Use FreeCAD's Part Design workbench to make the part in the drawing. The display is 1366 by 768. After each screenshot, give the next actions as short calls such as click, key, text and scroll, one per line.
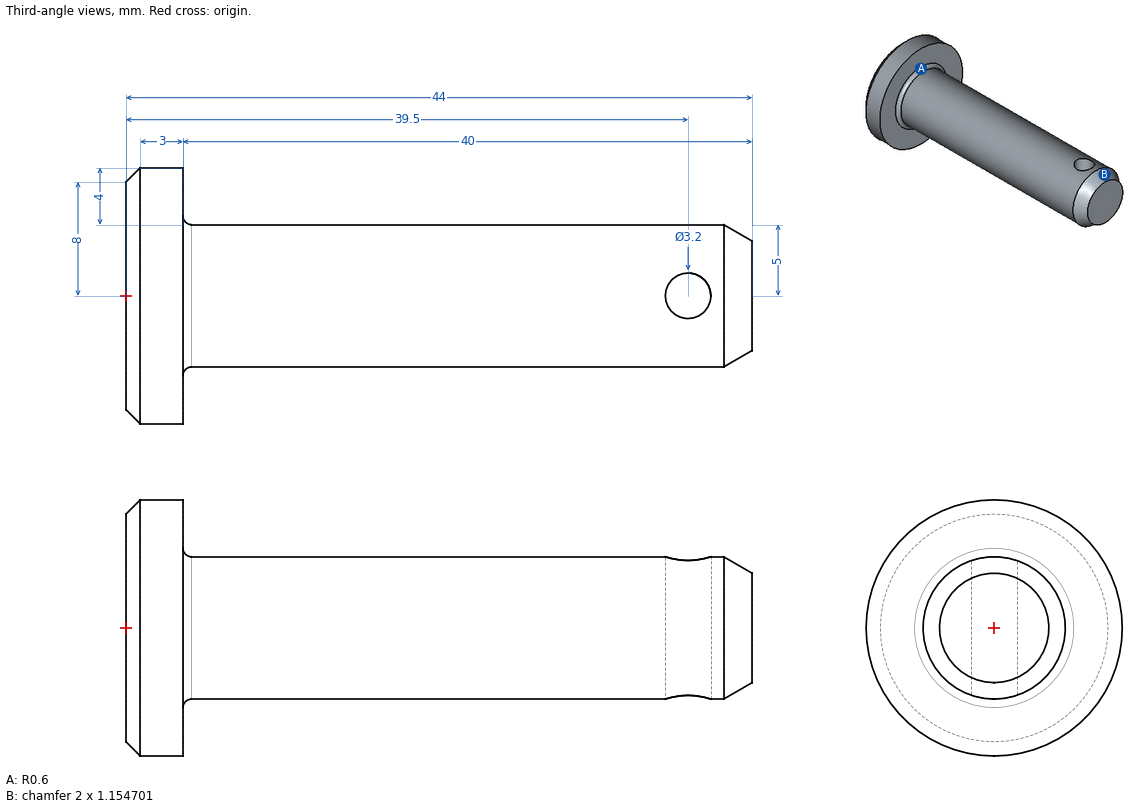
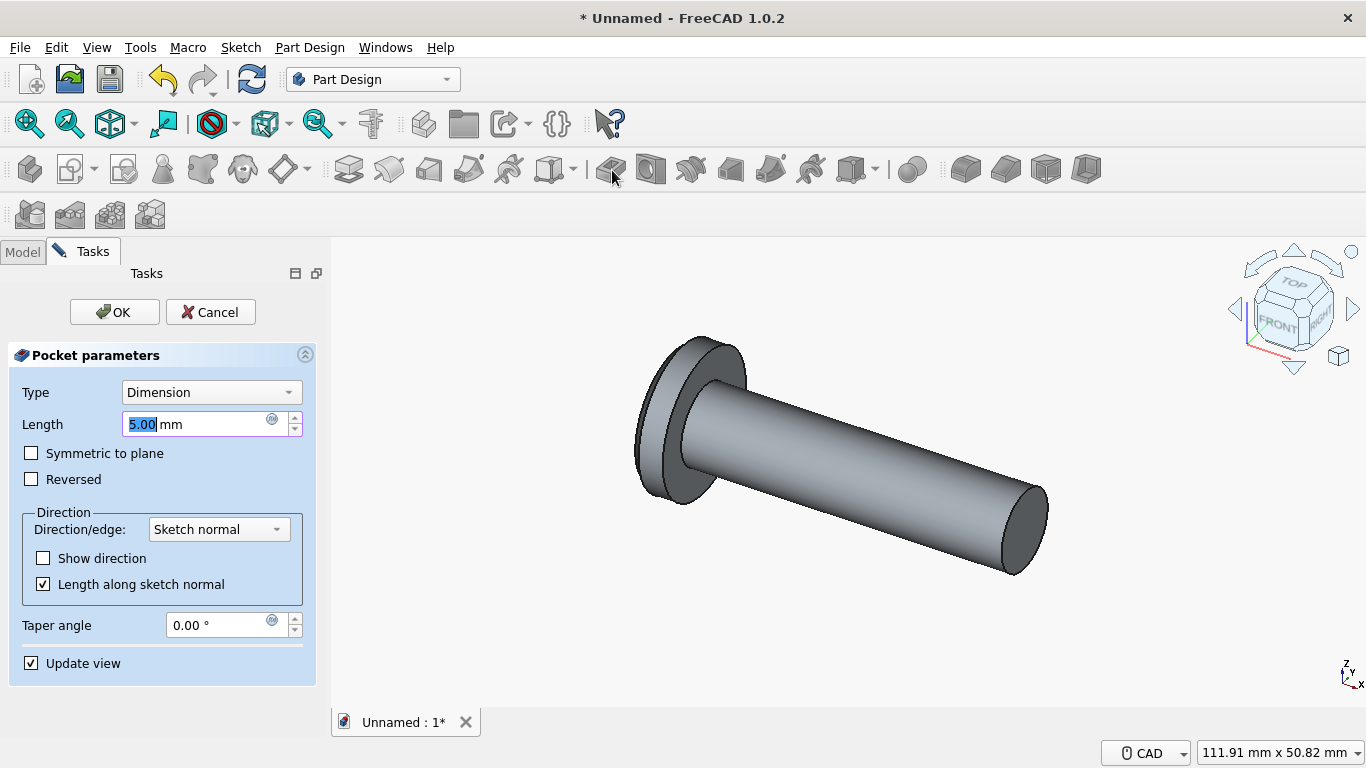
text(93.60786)
key(Tab)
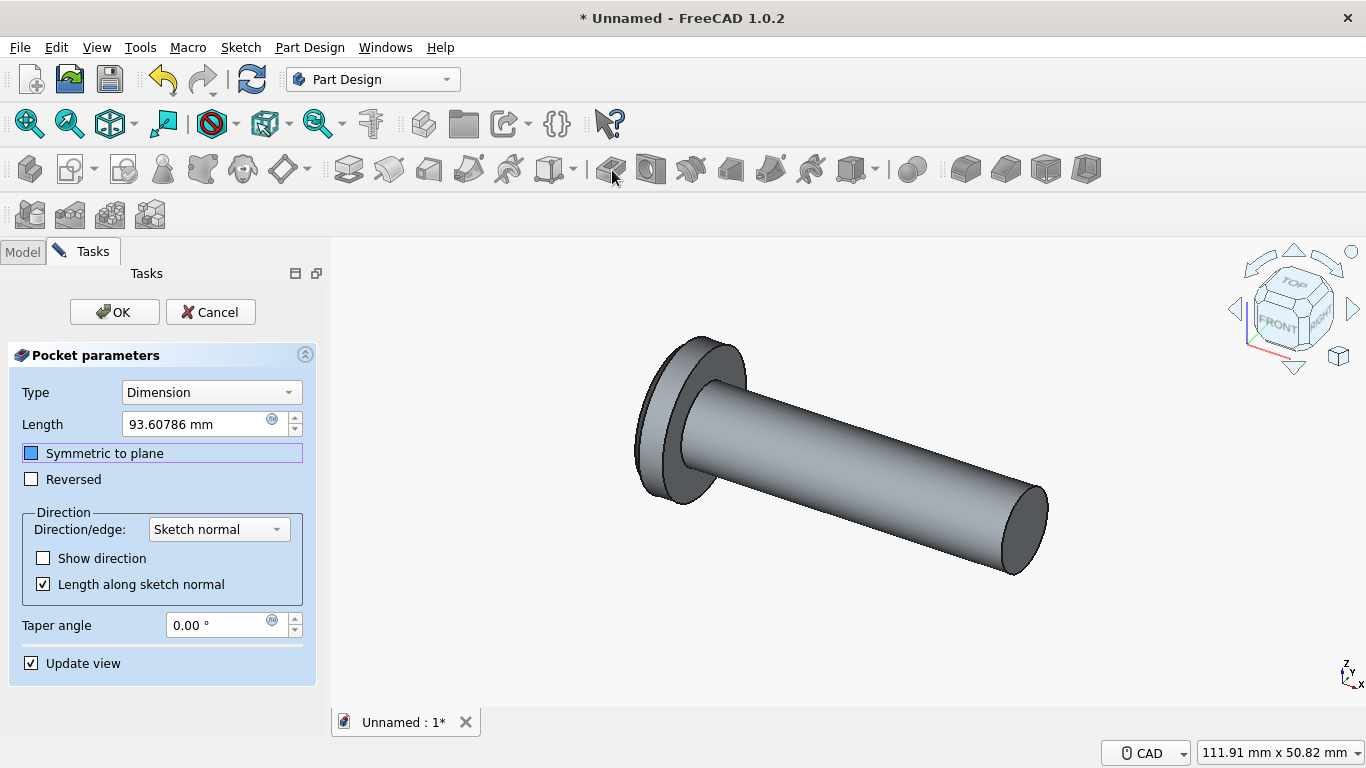
click(30, 453)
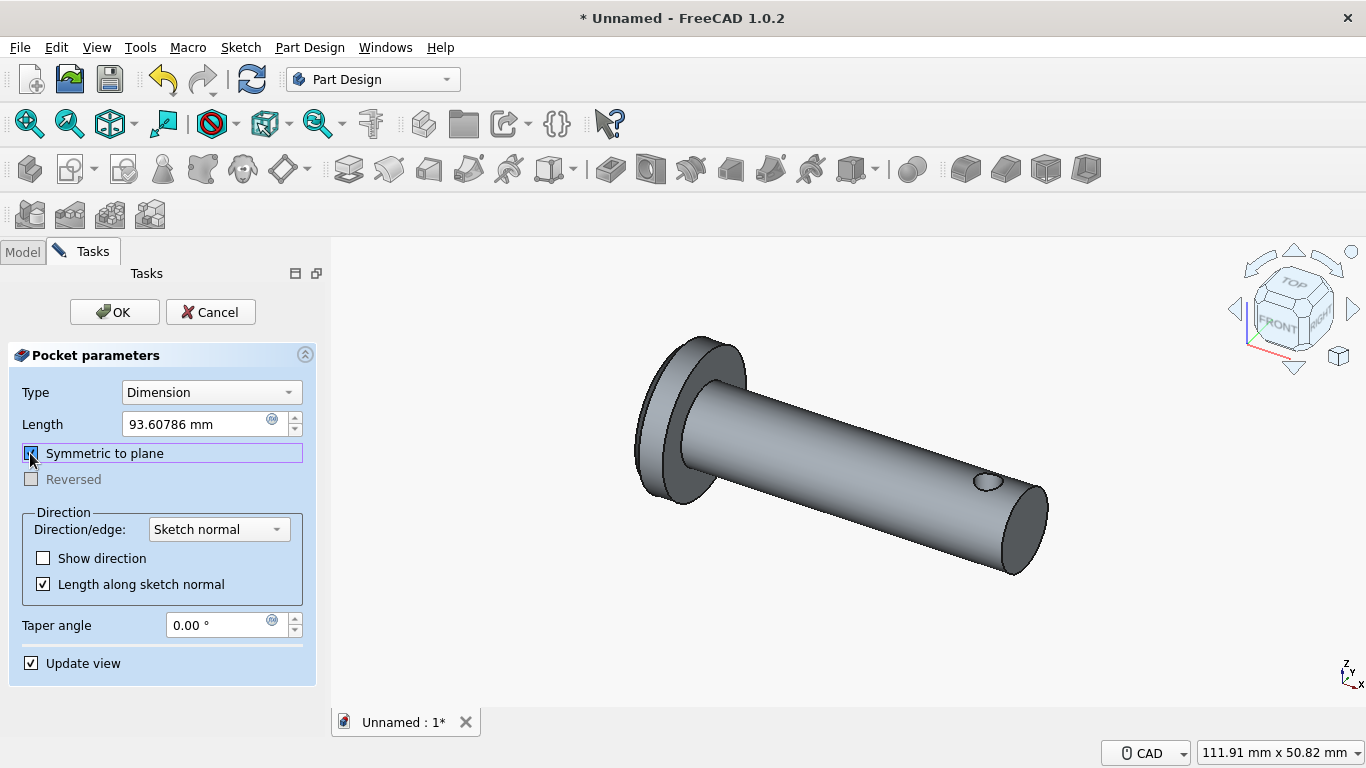
click(115, 312)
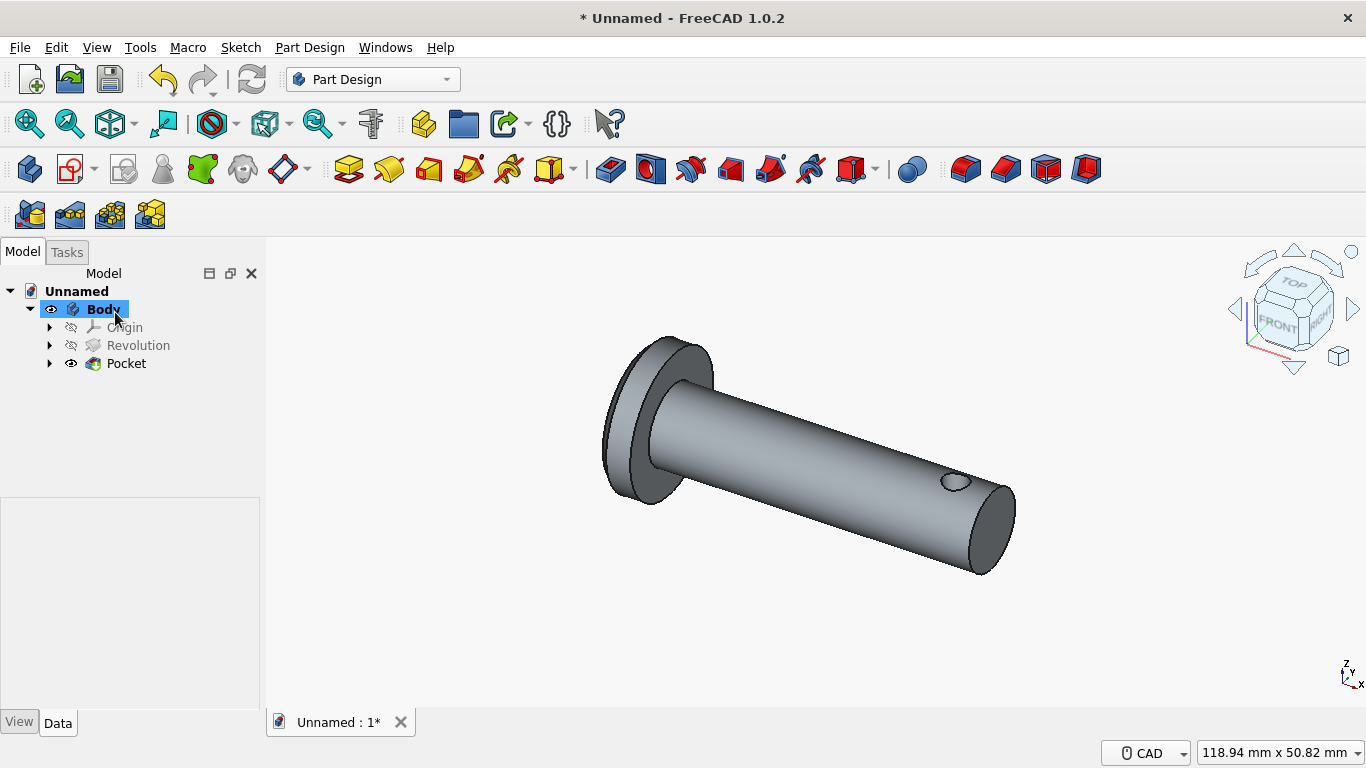
key(0)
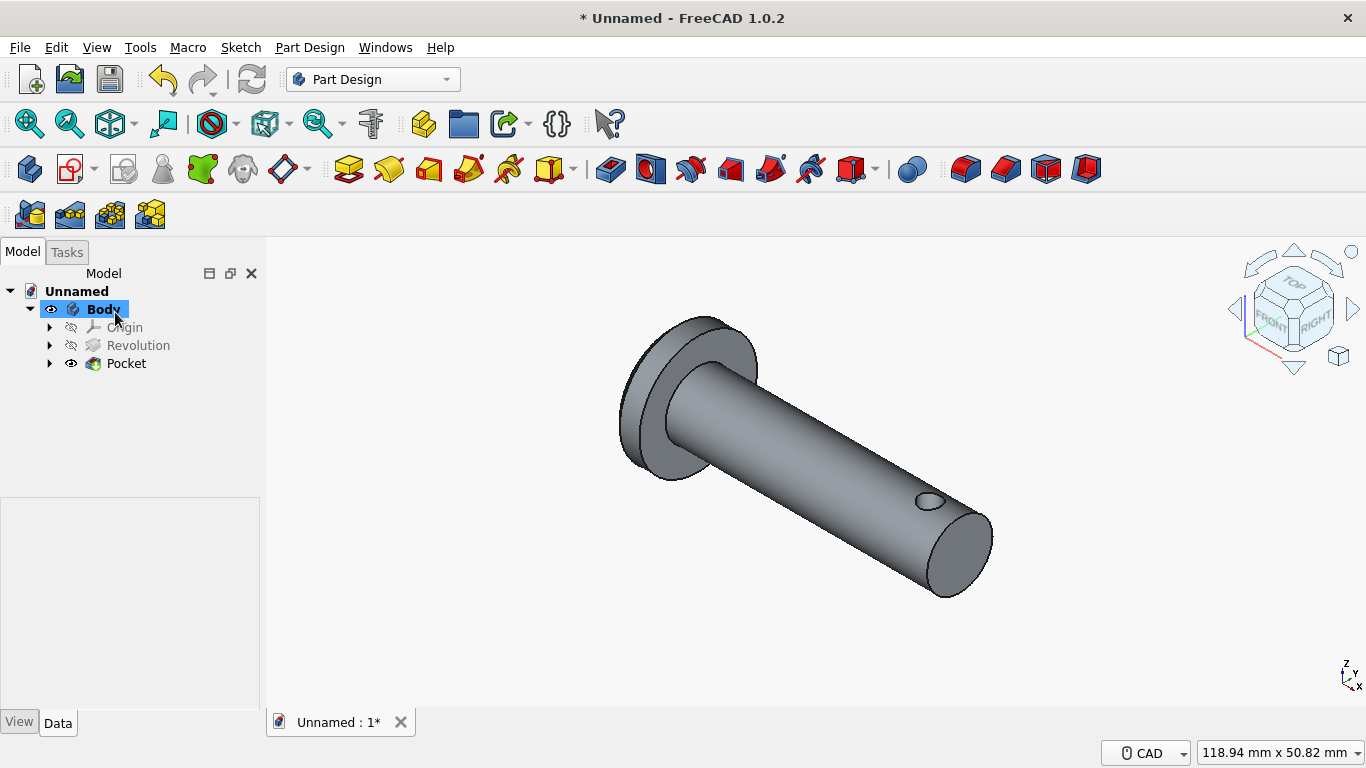
key(2)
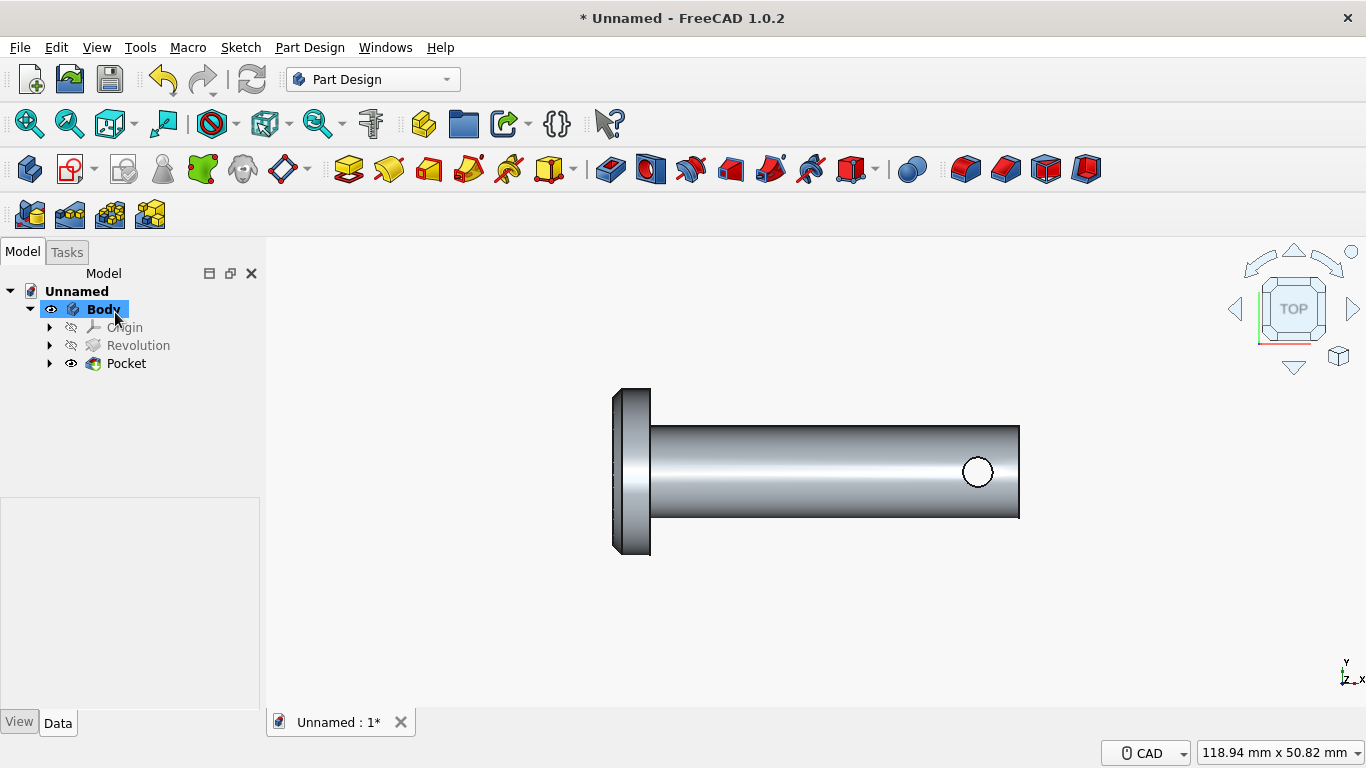
click(30, 124)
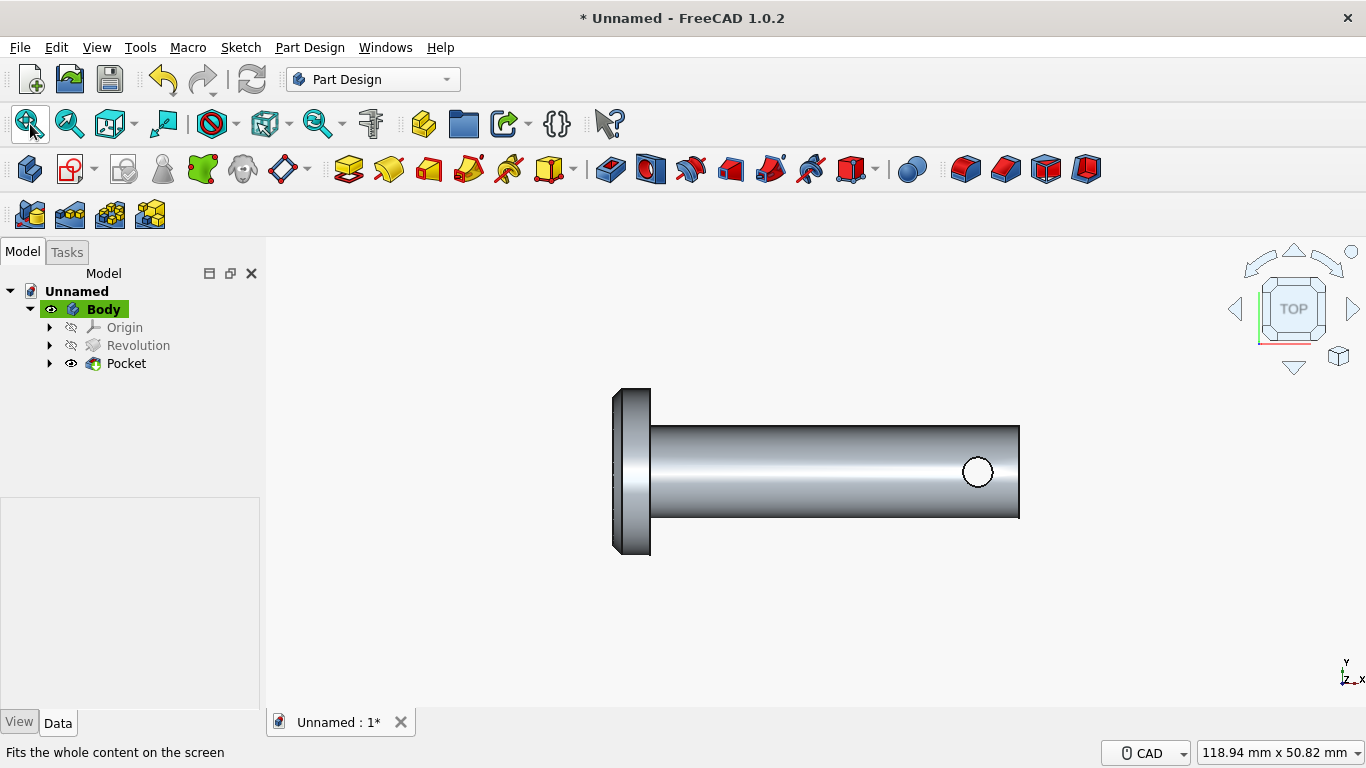
key(1)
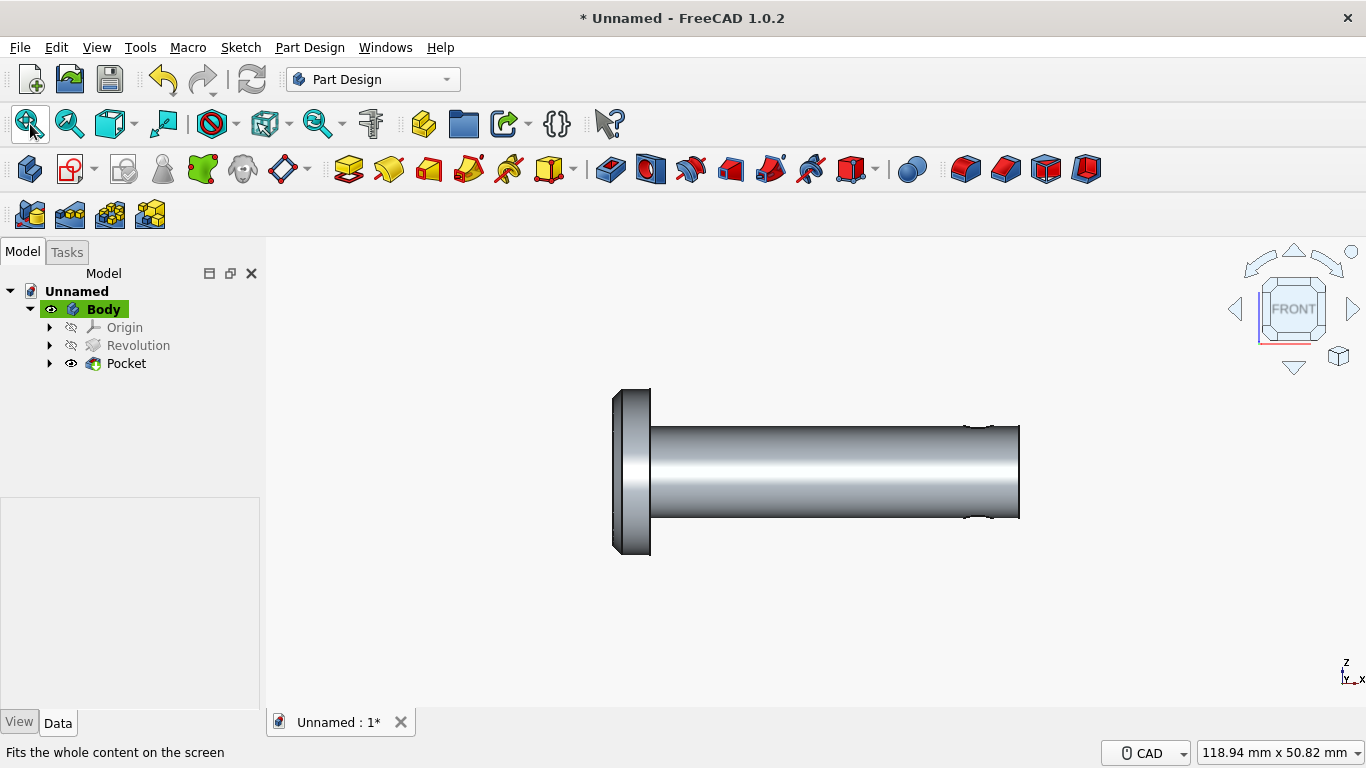
click(30, 124)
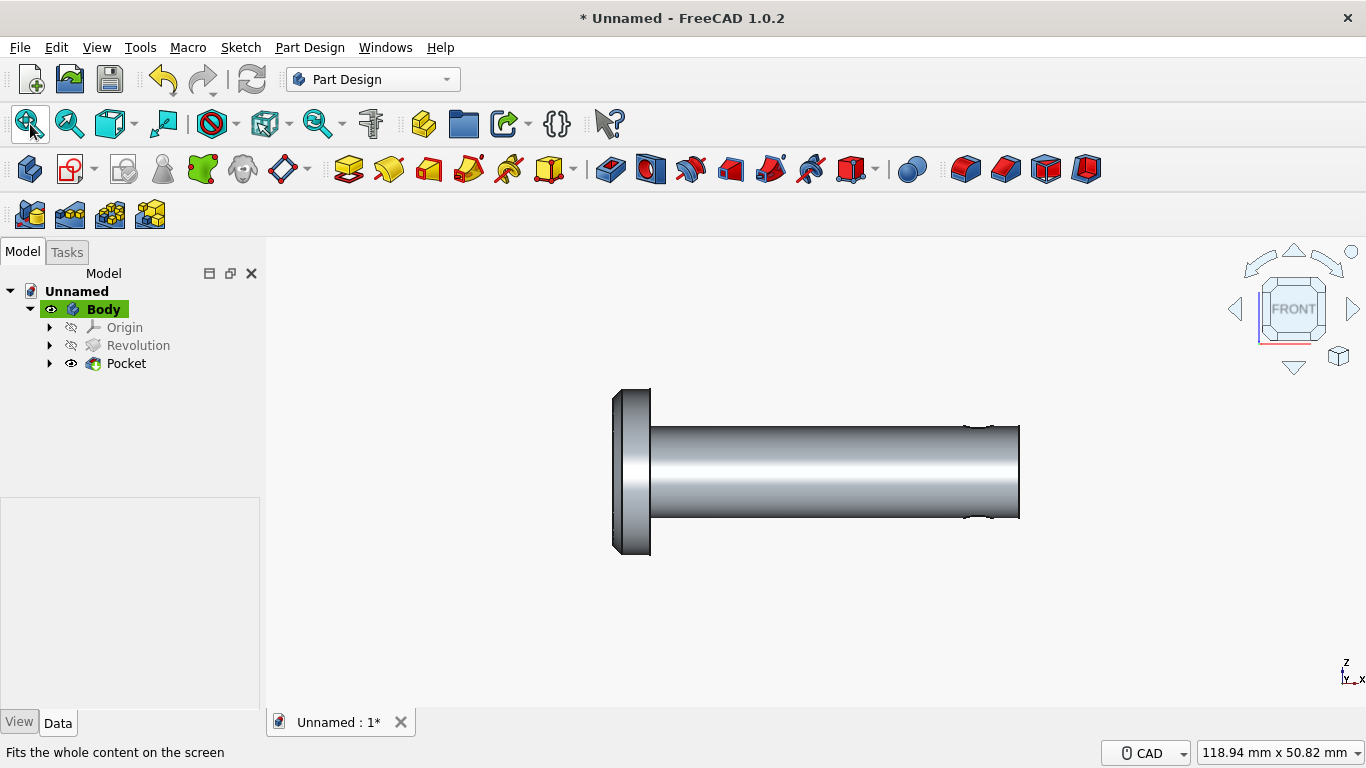
key(3)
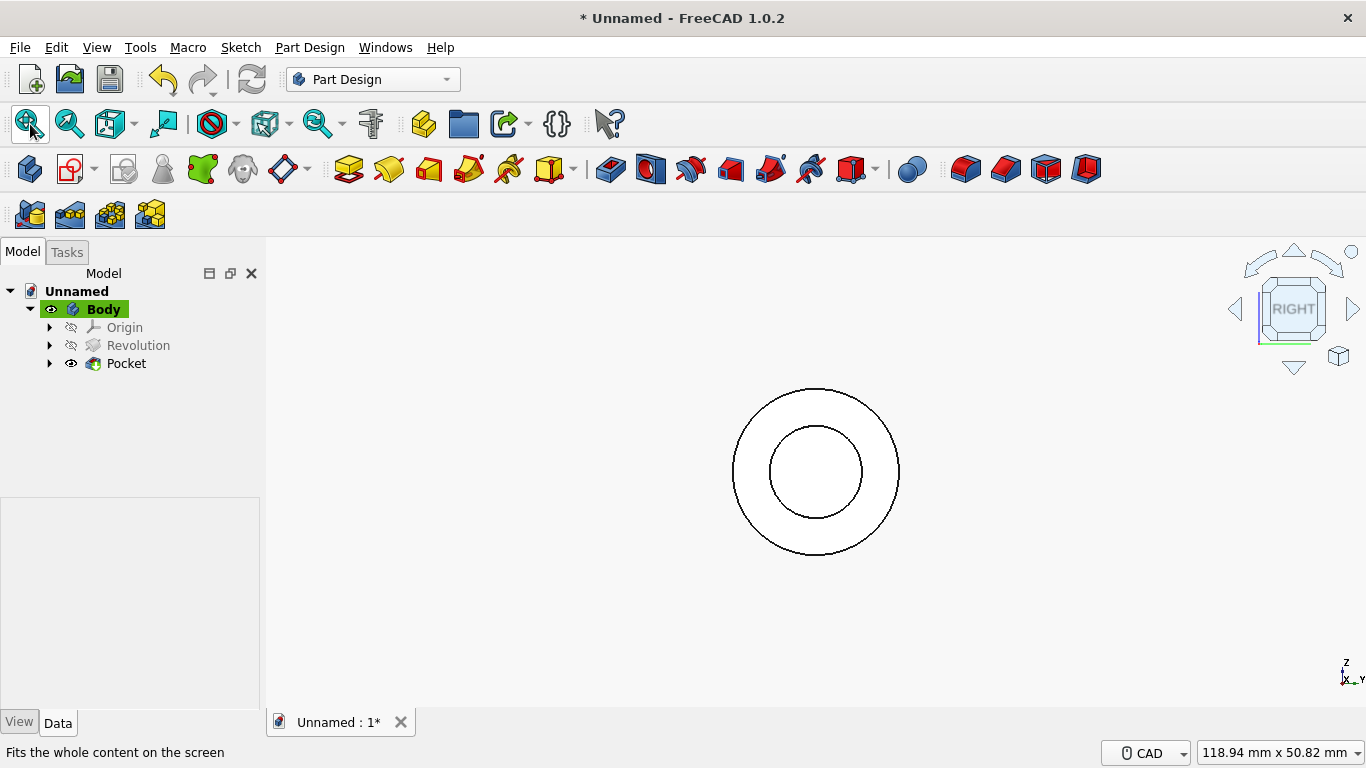
click(30, 124)